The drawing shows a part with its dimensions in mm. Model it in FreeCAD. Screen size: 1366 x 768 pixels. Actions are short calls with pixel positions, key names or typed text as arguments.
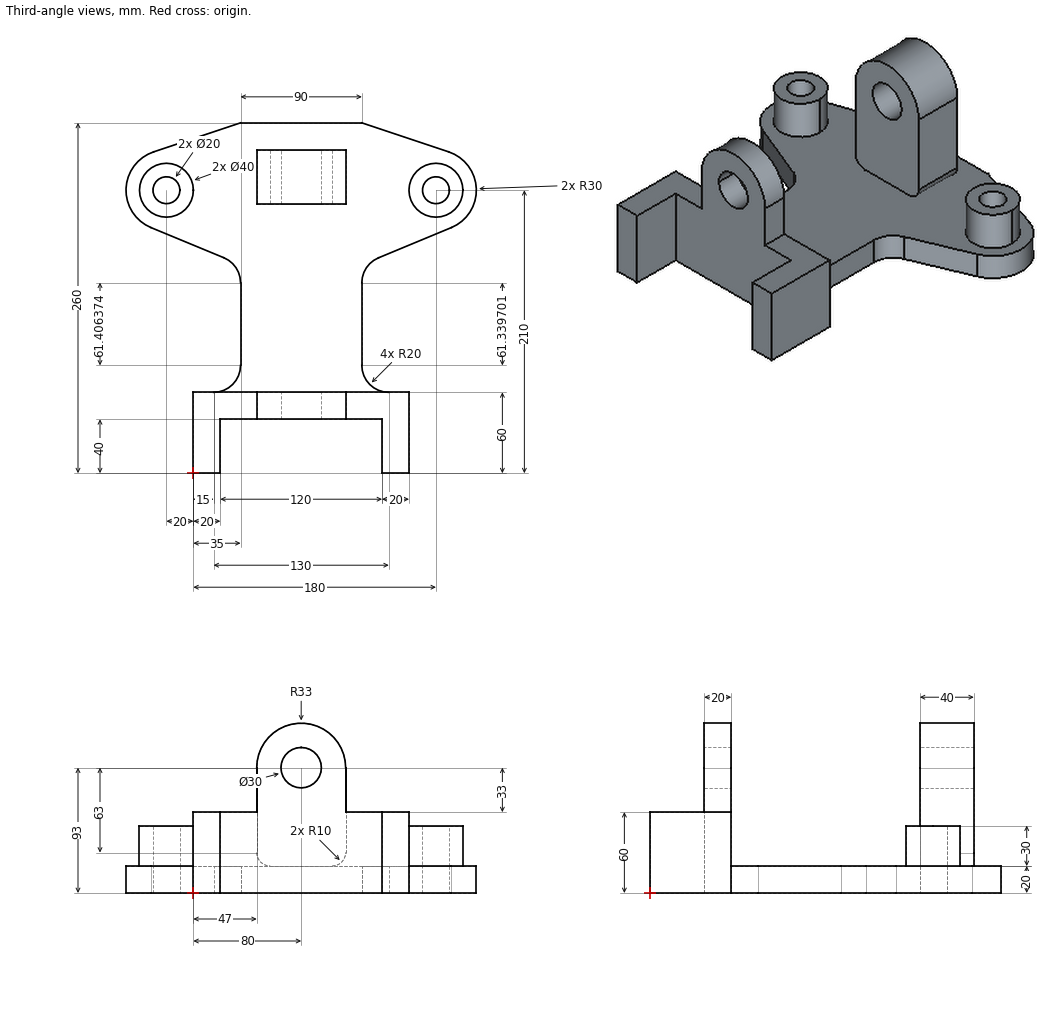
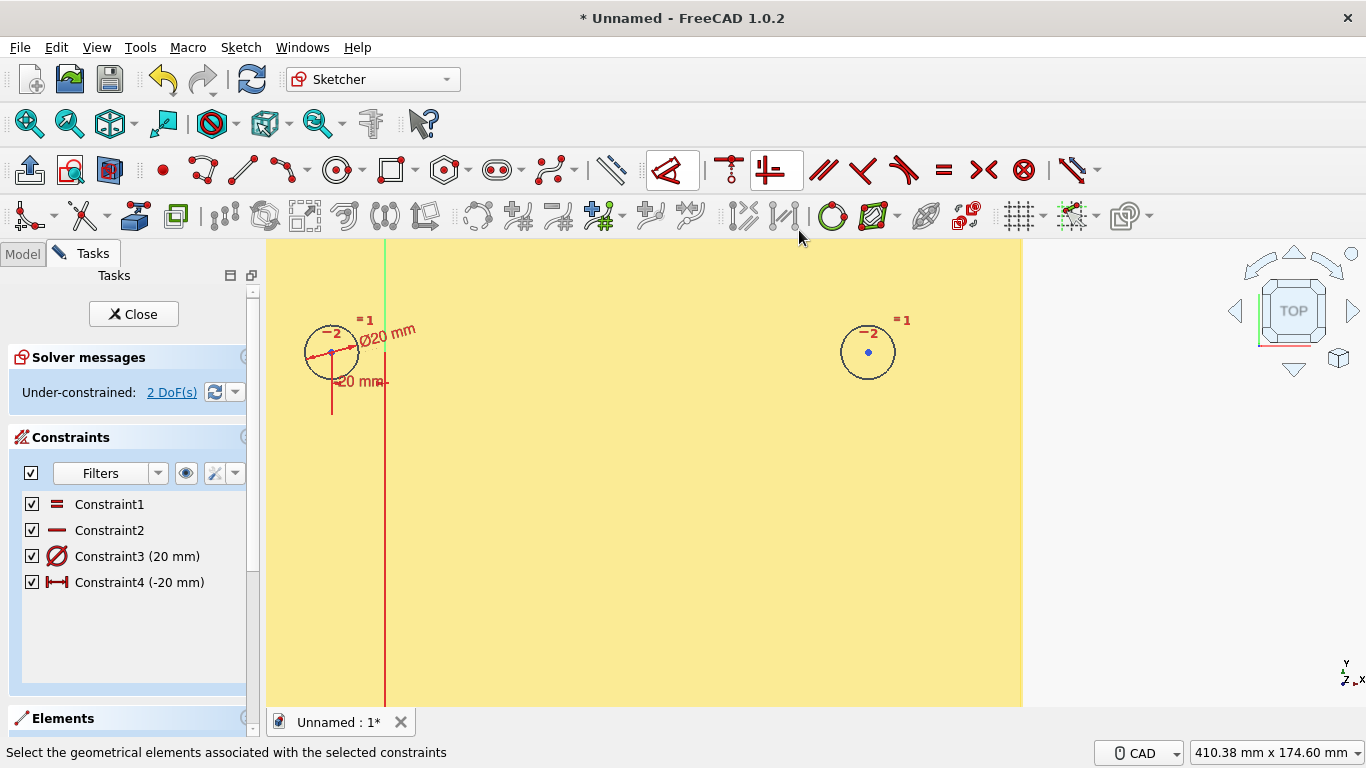
click(332, 352)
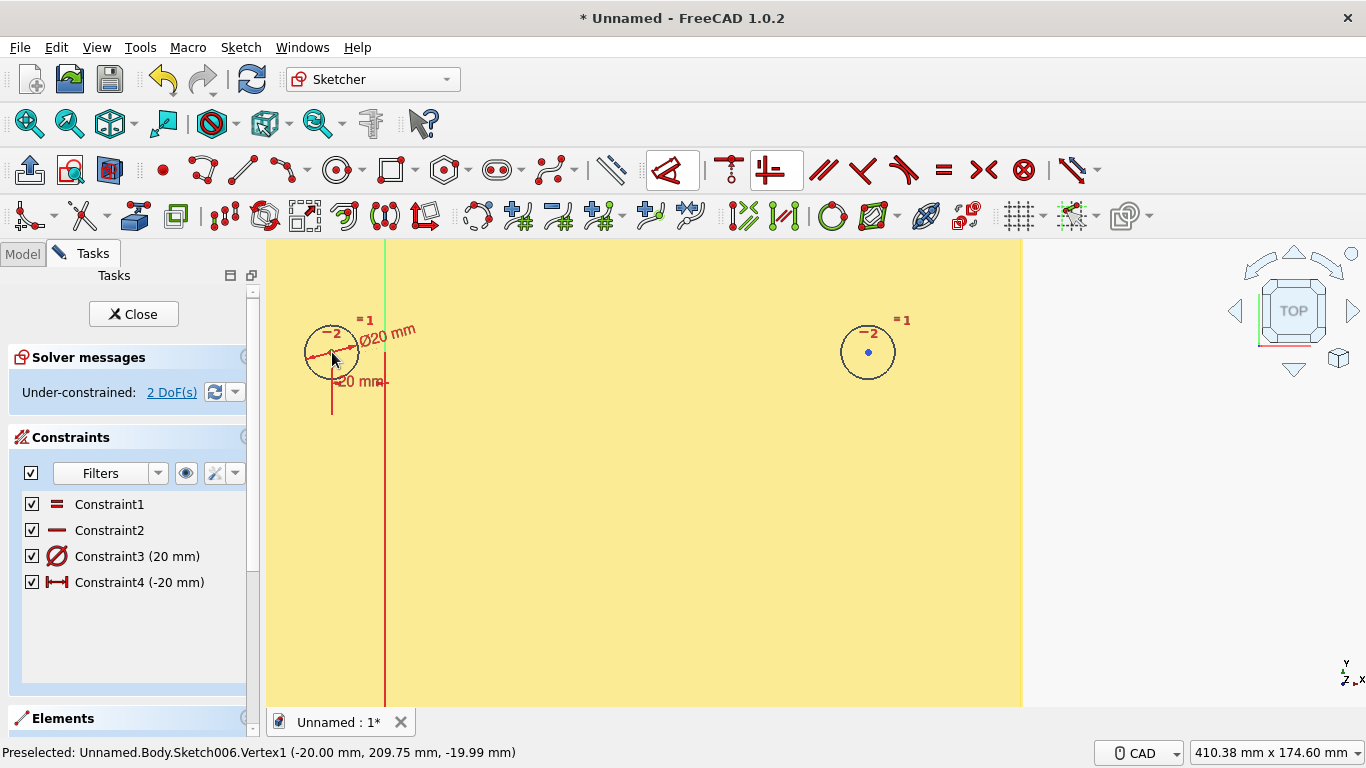
key(i)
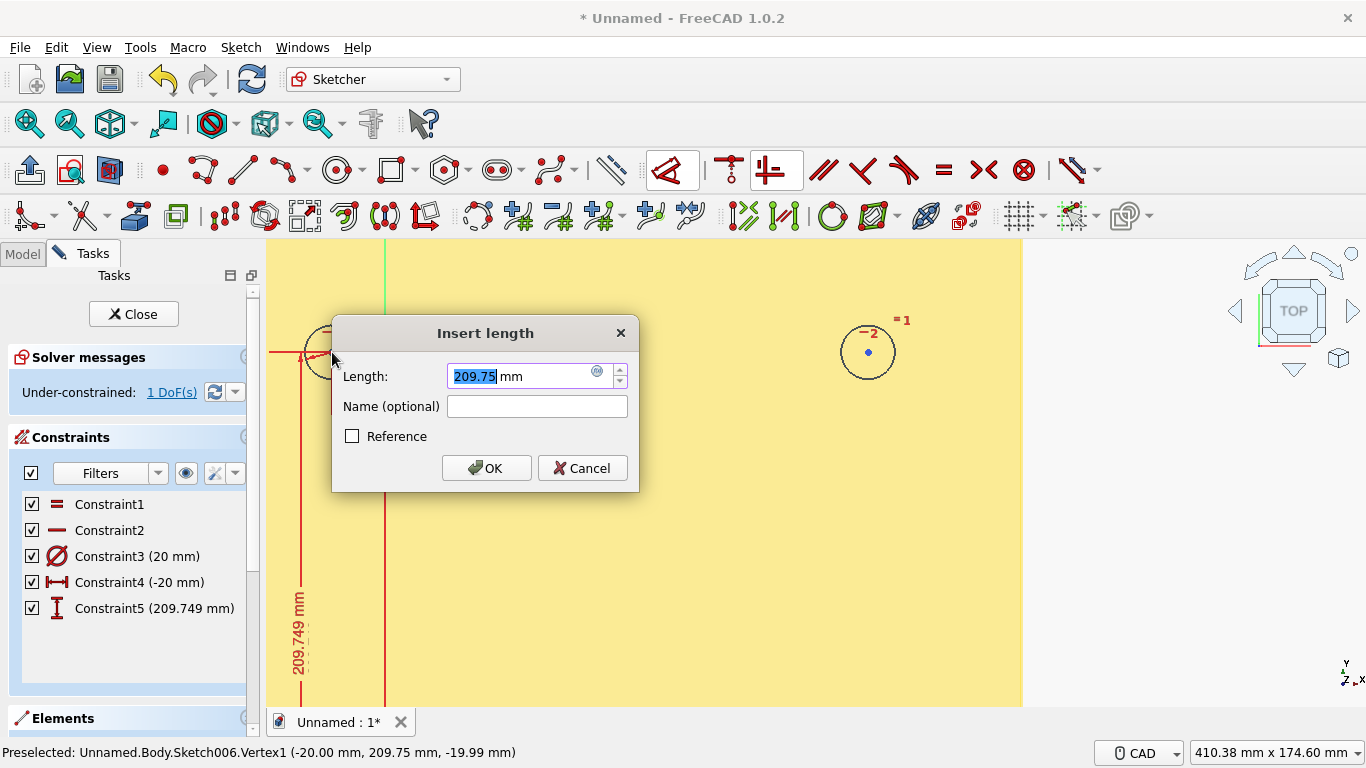
text(210)
key(Return)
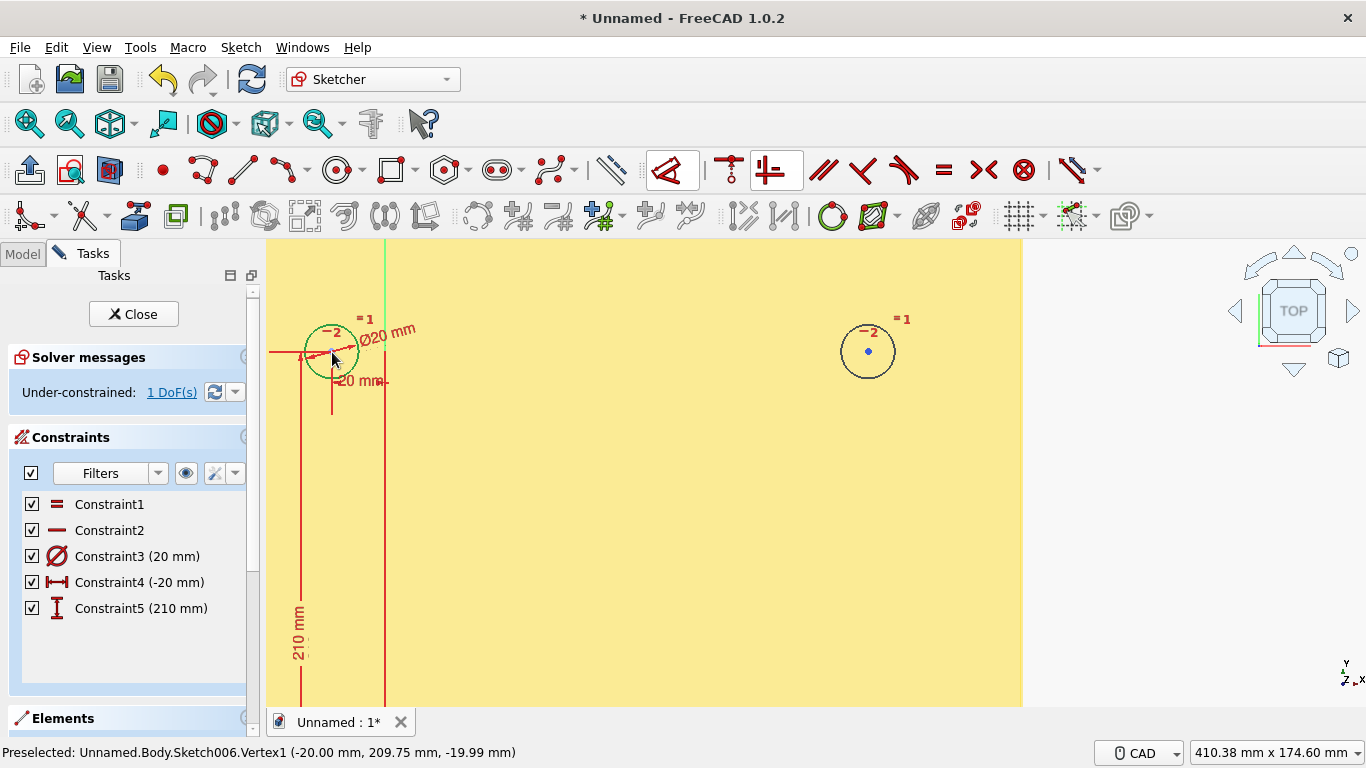
click(868, 352)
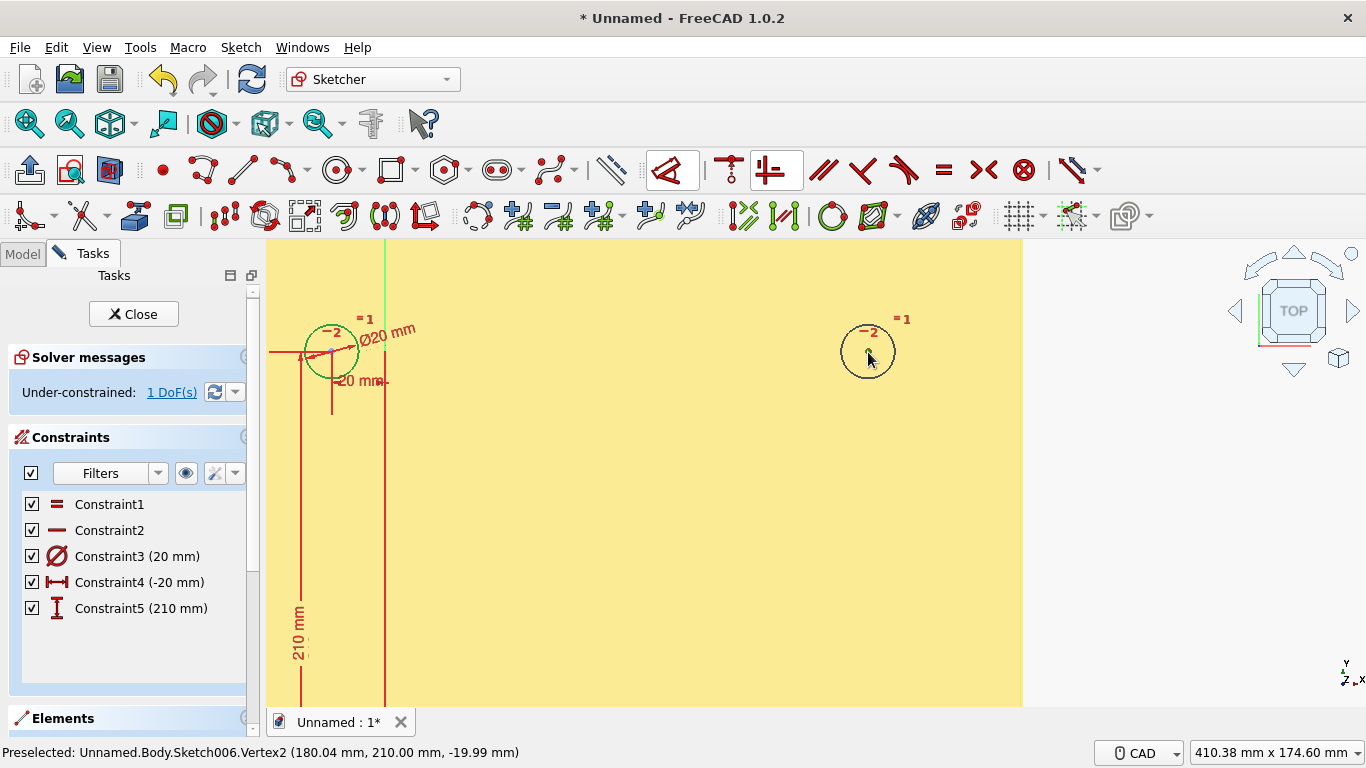
click(694, 170)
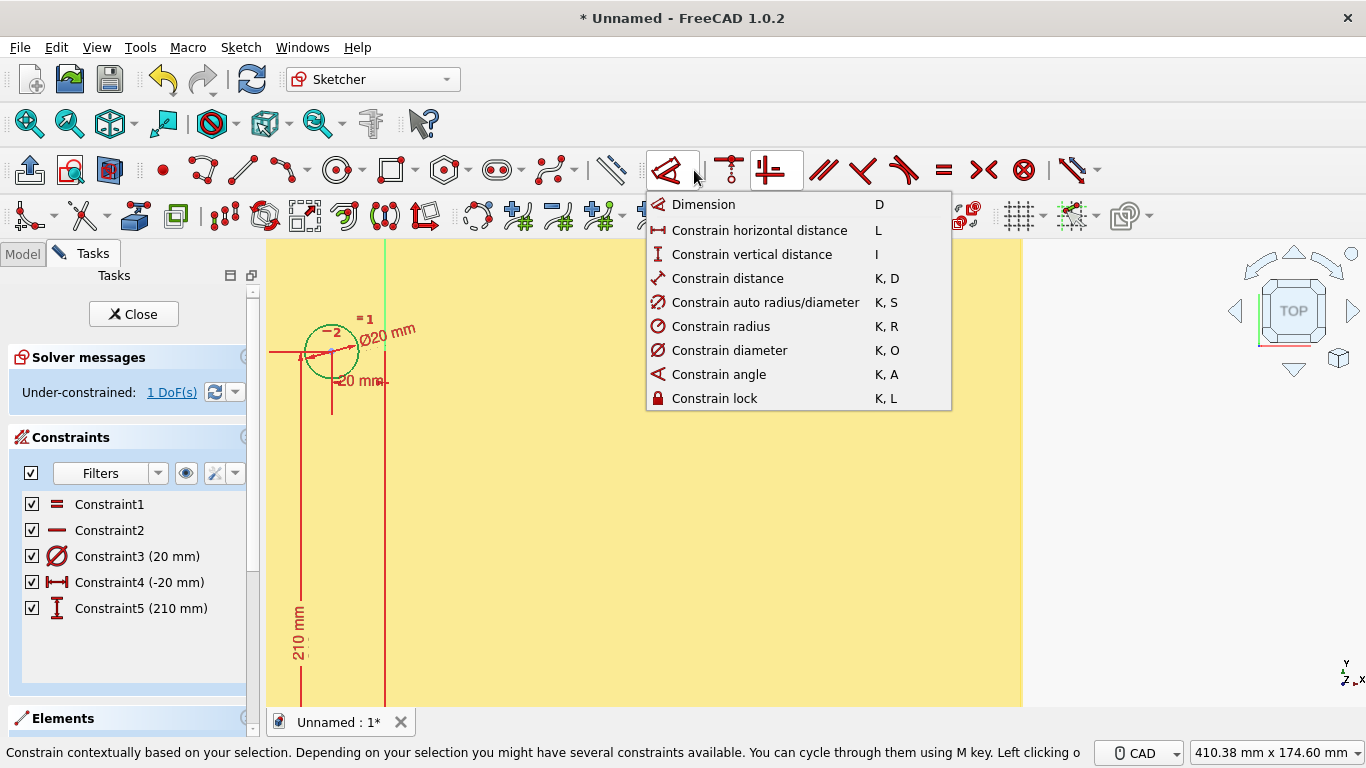
click(799, 230)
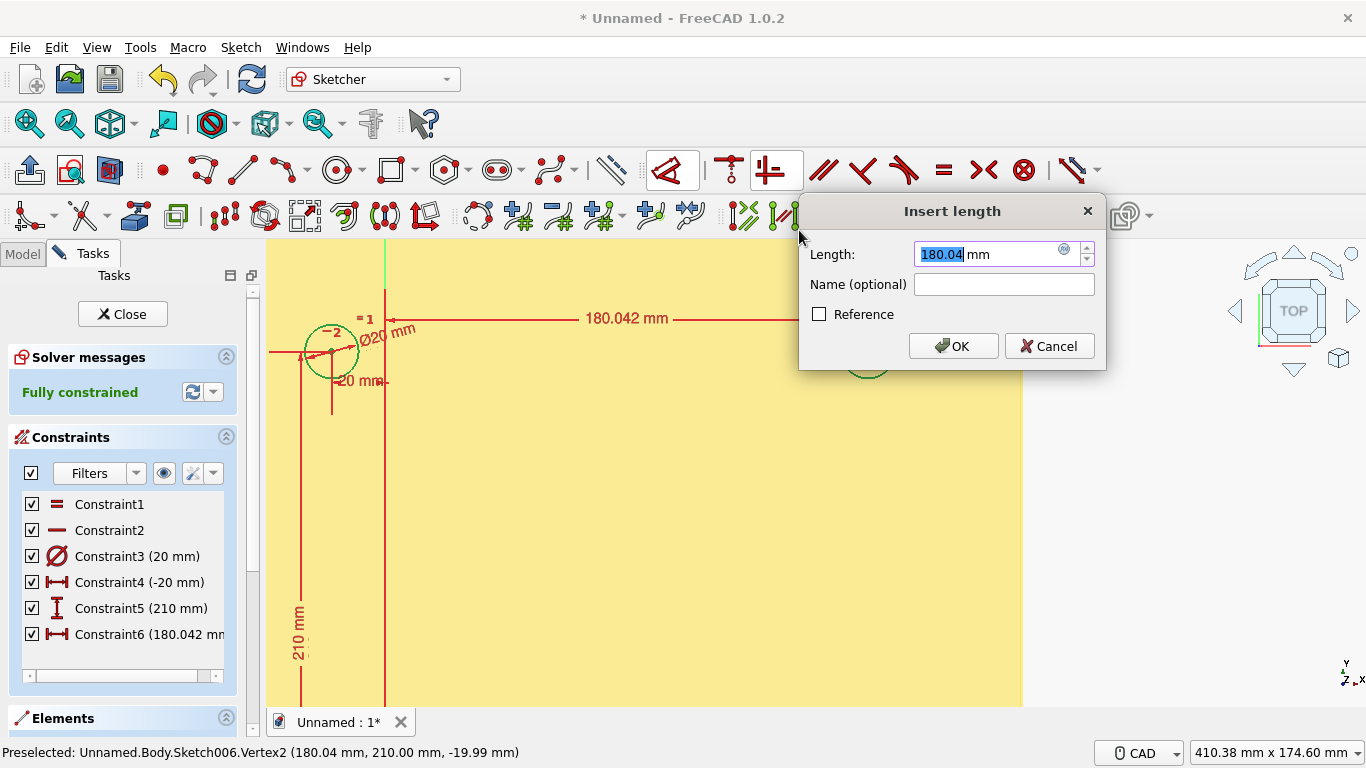
text(180)
key(Return)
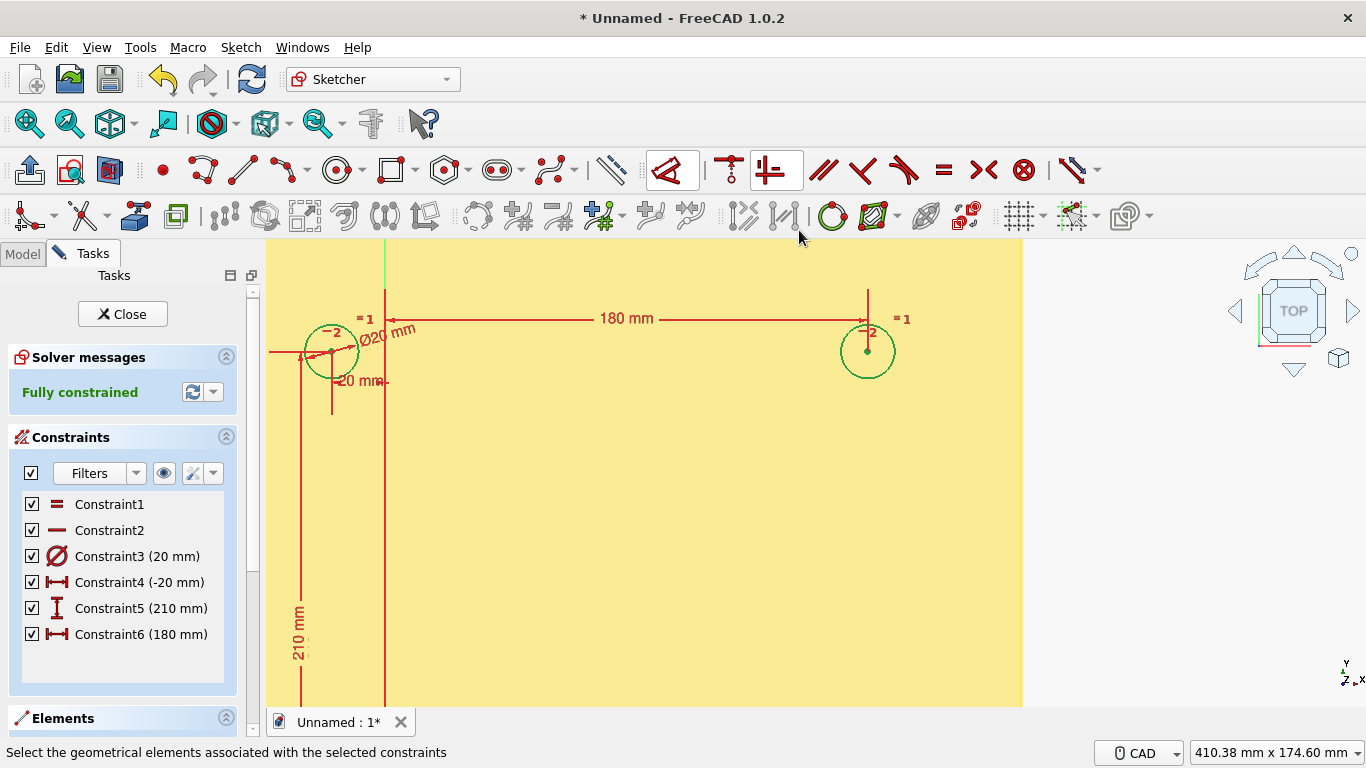
click(123, 314)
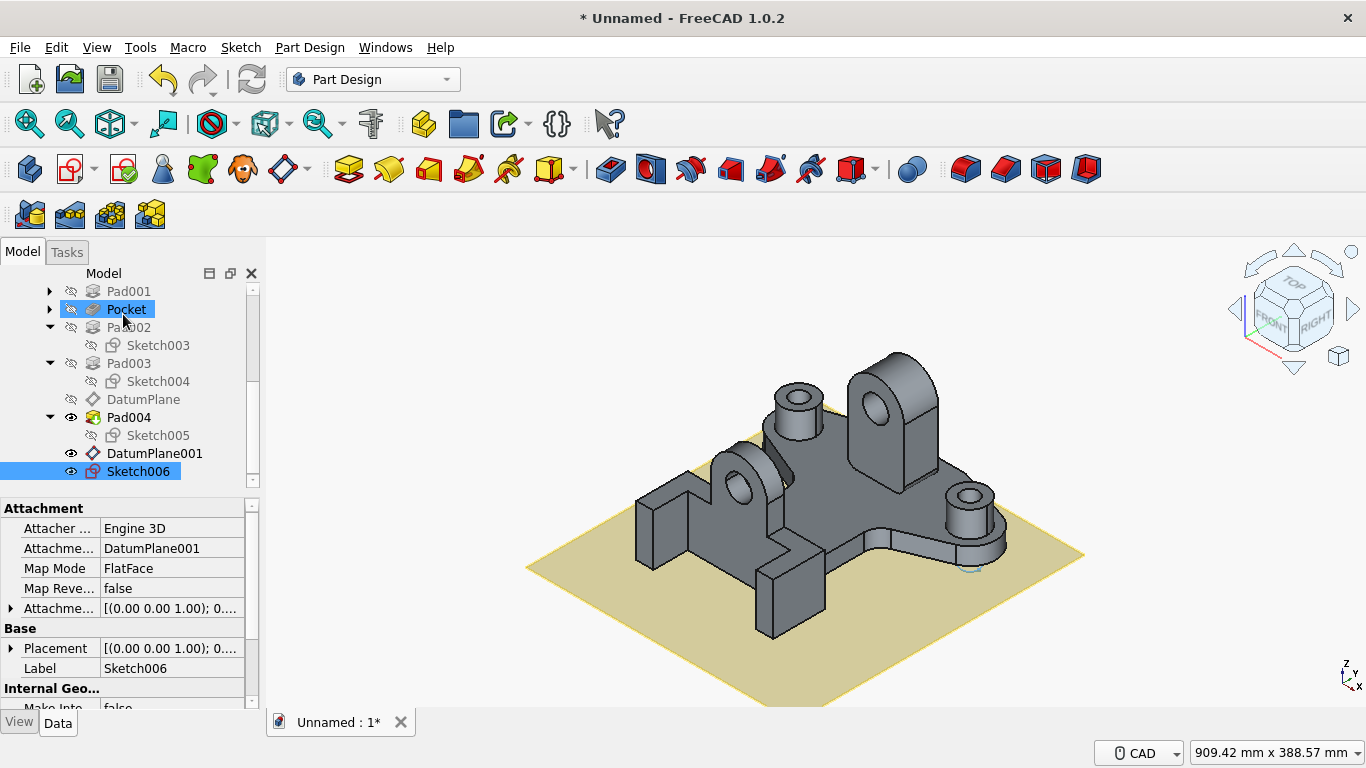
click(612, 170)